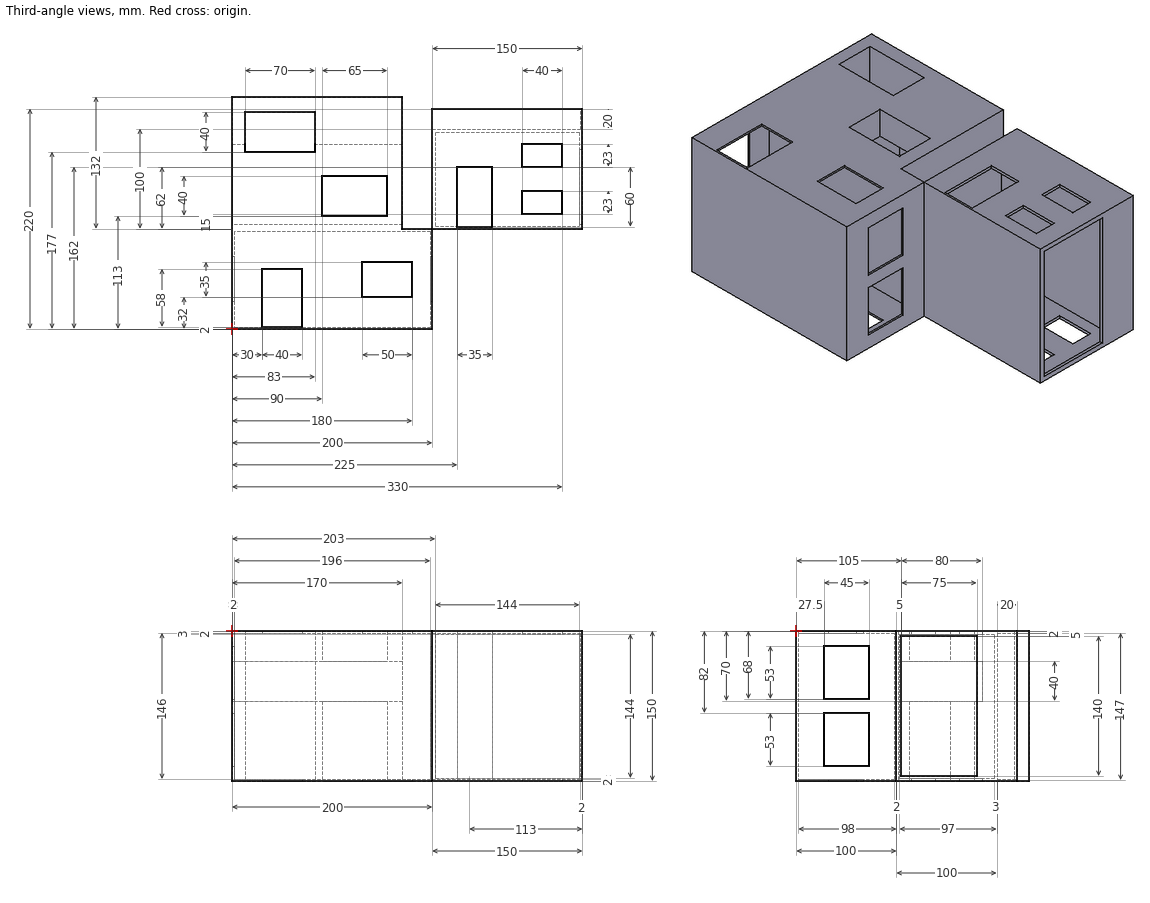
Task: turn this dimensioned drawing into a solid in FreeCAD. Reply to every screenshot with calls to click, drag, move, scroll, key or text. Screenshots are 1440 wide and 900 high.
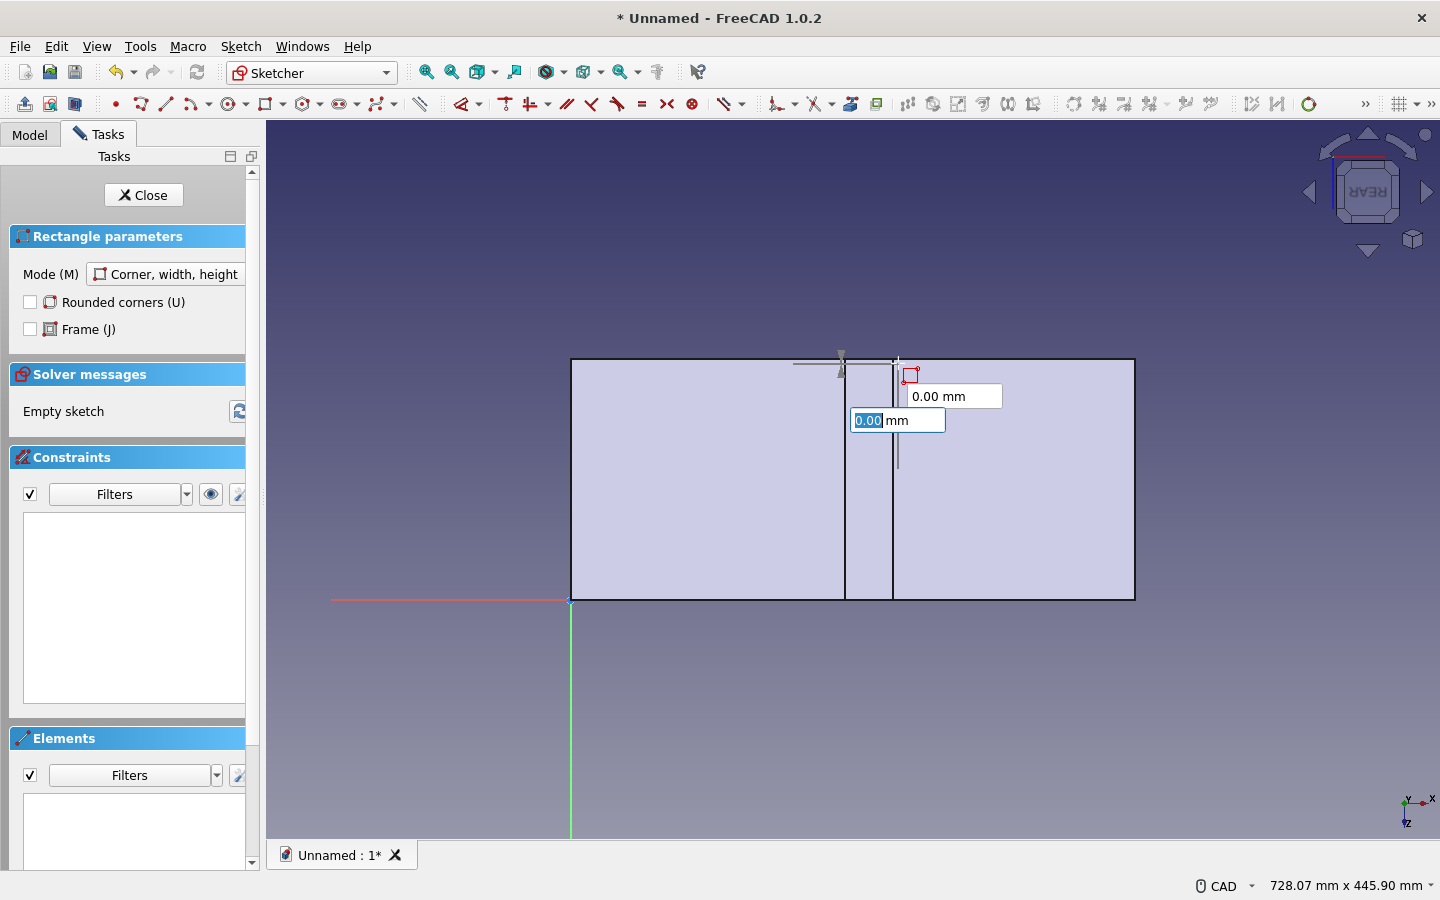
scroll(1130, 596, up, 6)
move(1129, 593)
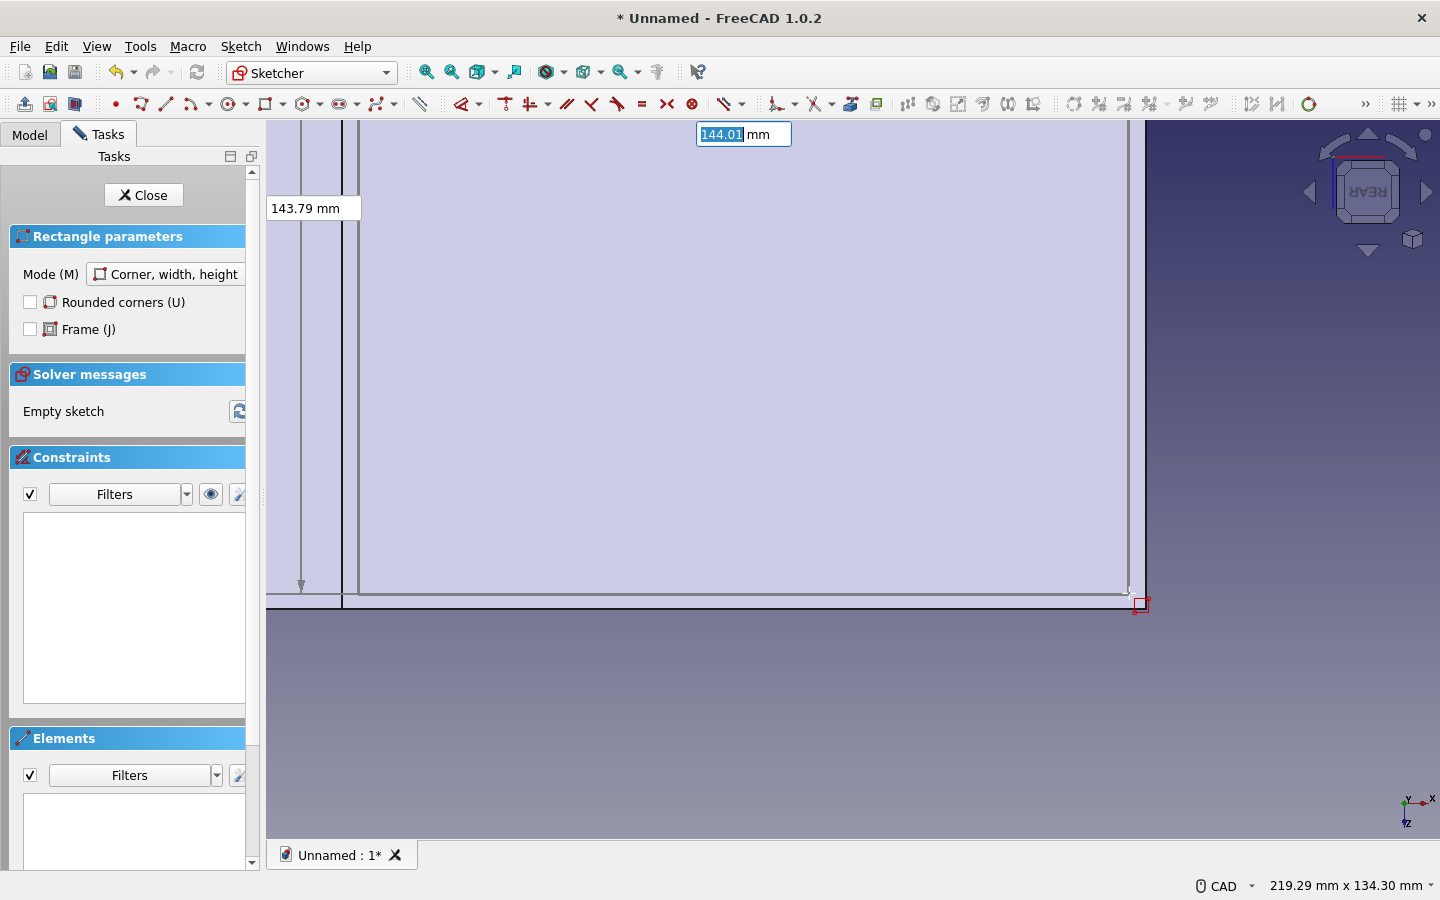
text(144)
key(Tab)
text(144)
key(Return)
key(Escape)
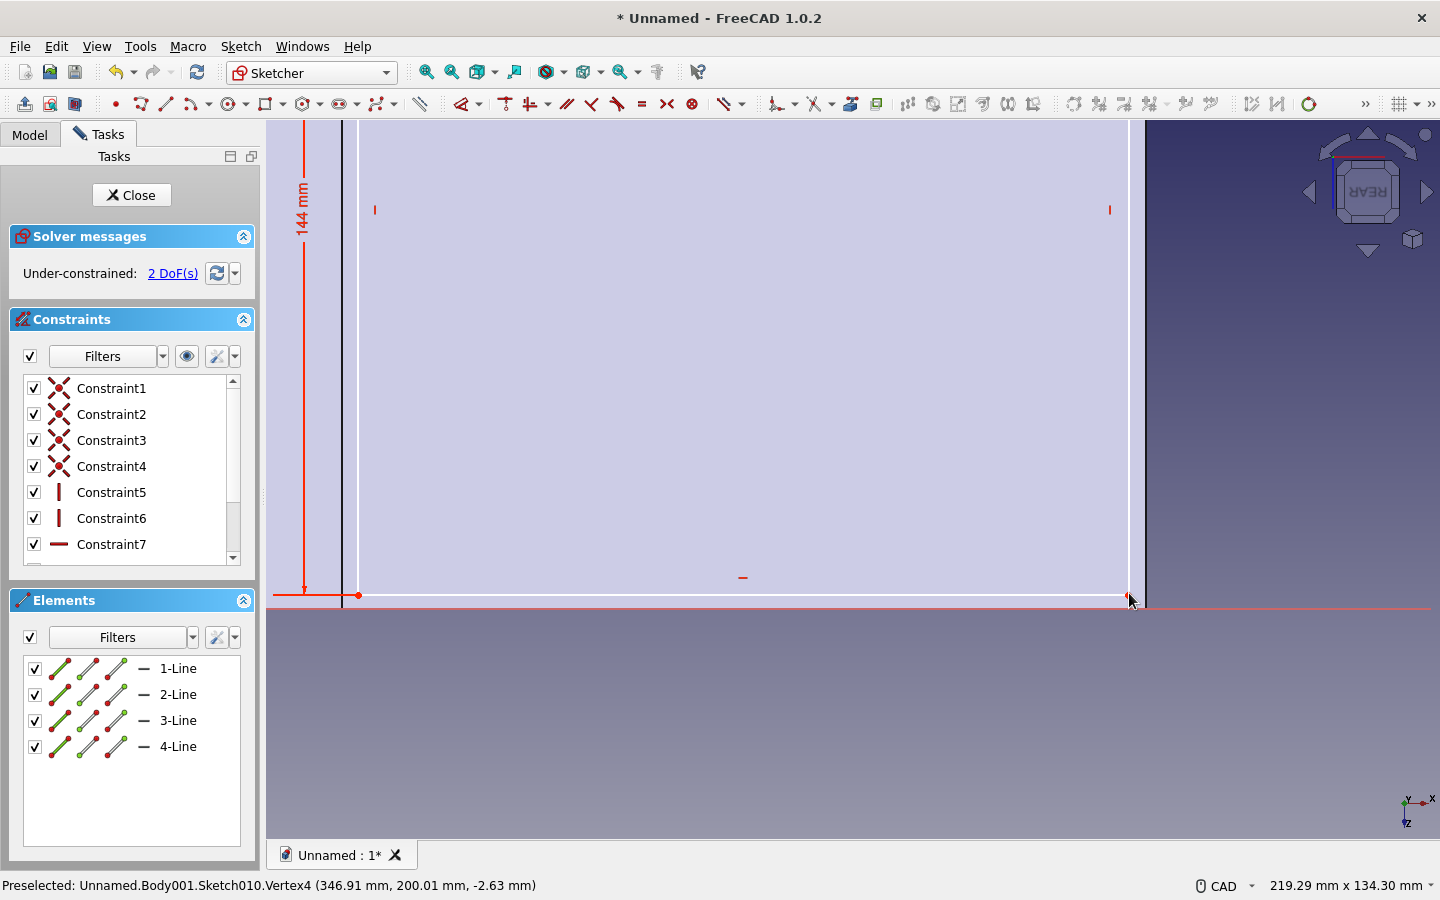
click(460, 104)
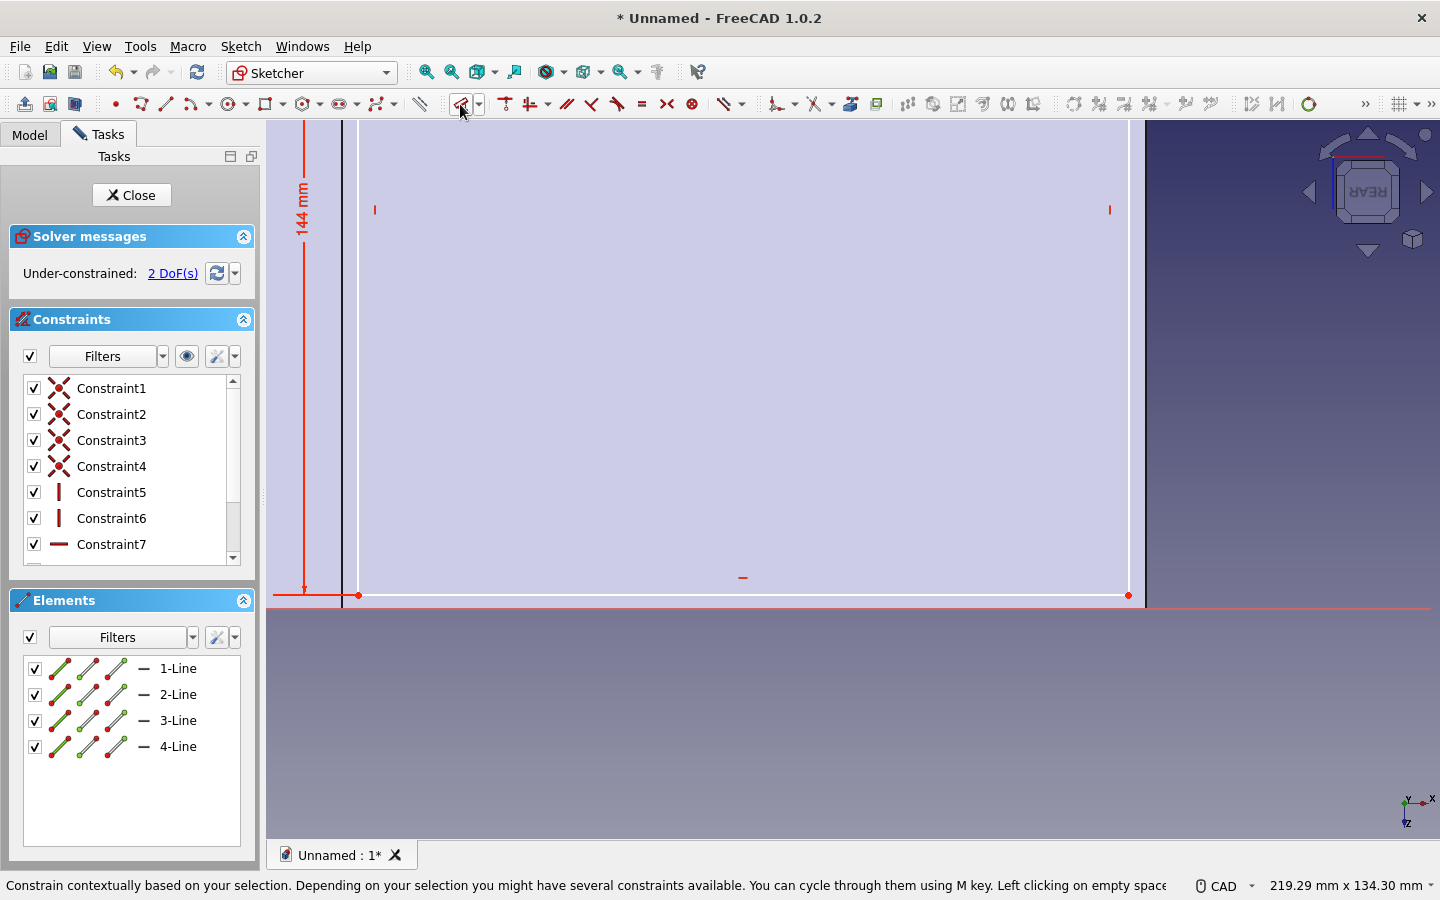
scroll(358, 595, up, 5)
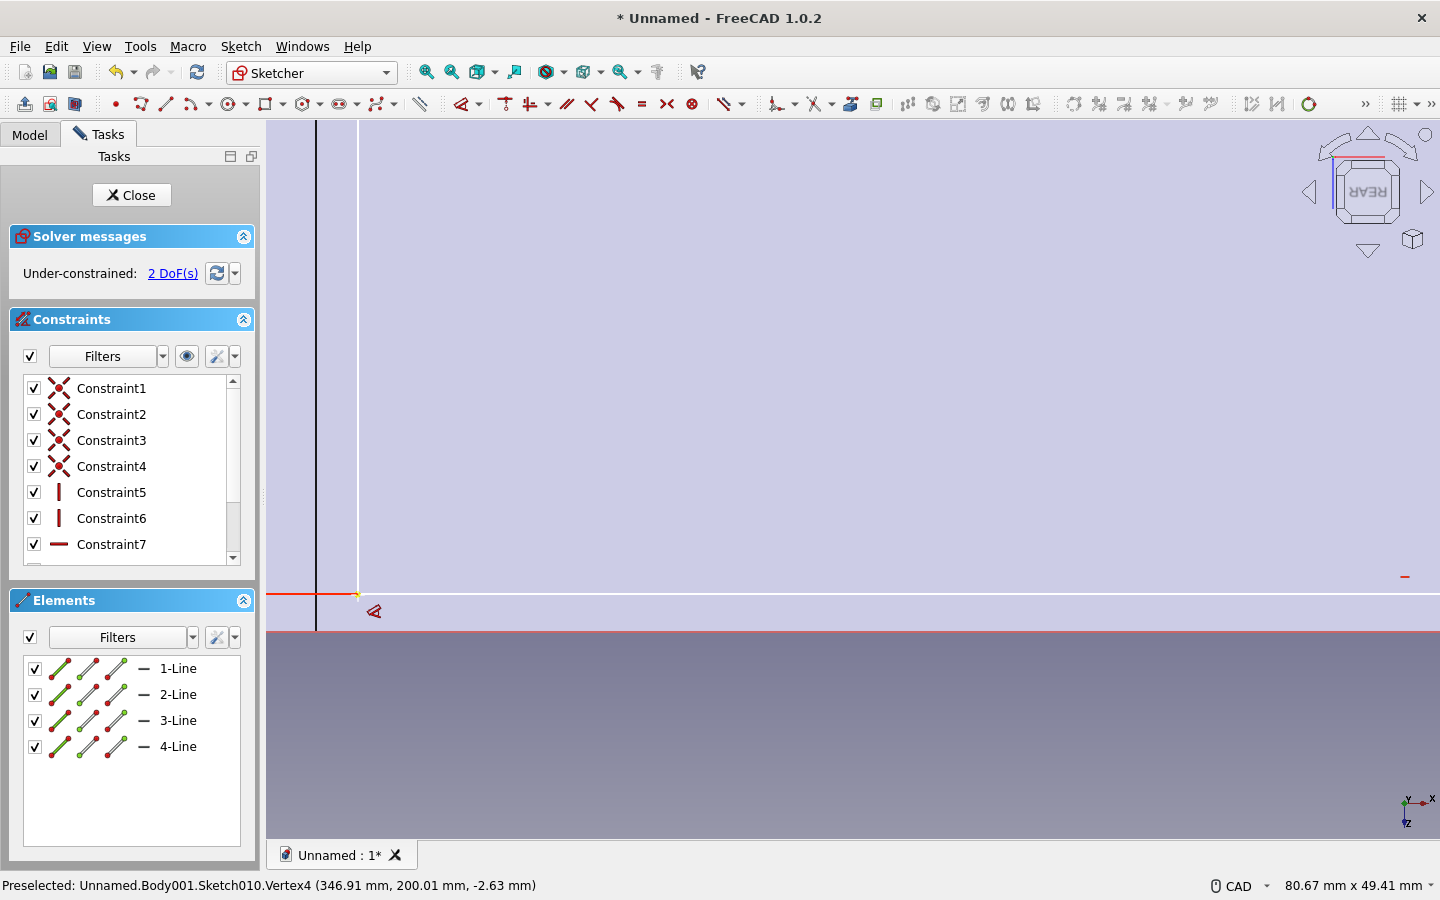
click(358, 594)
click(392, 613)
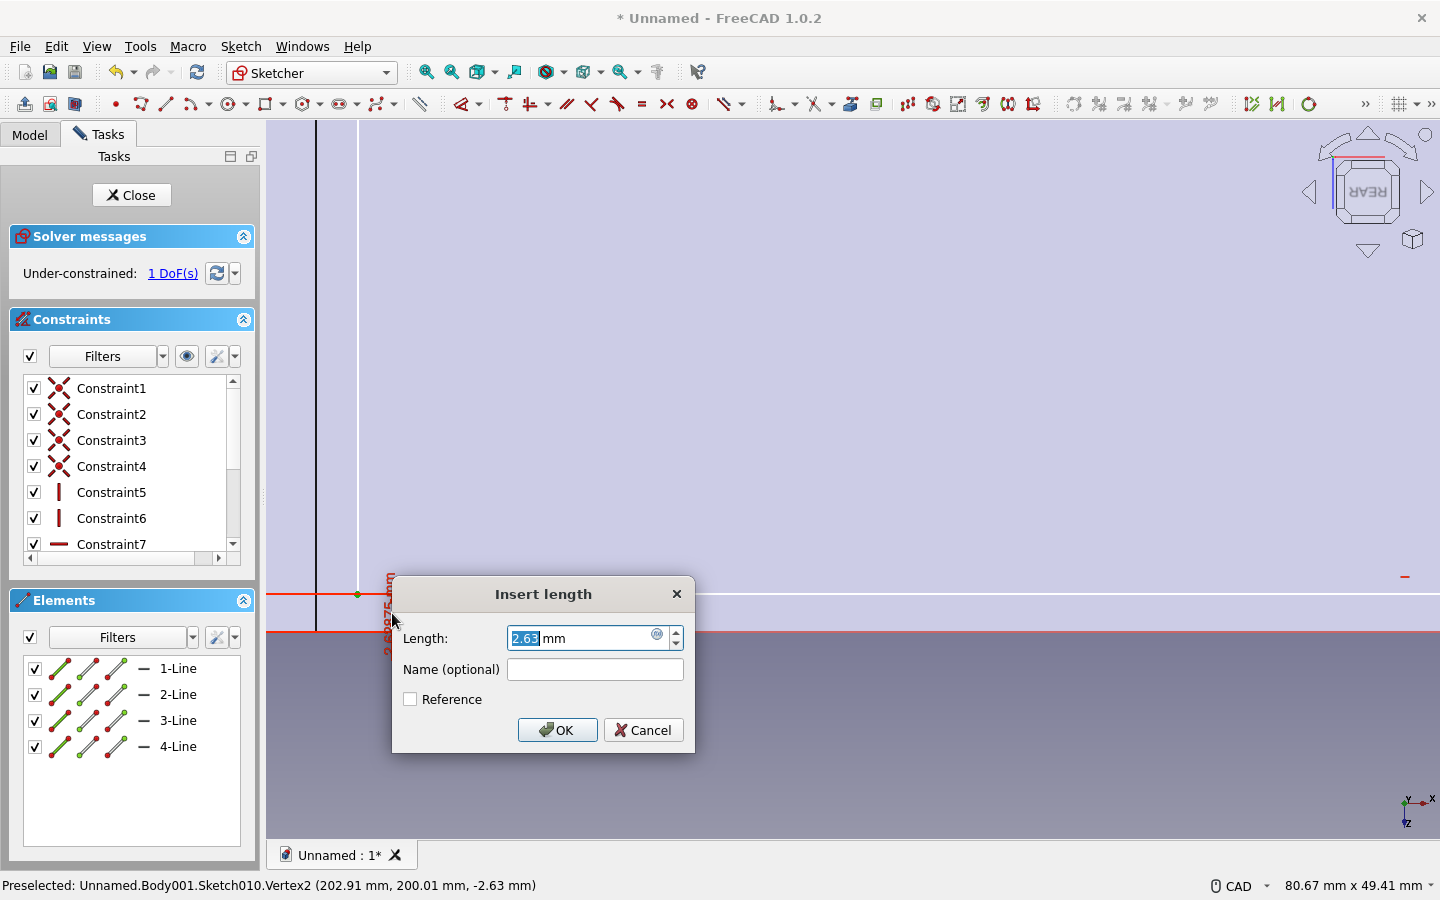
text(3)
key(Return)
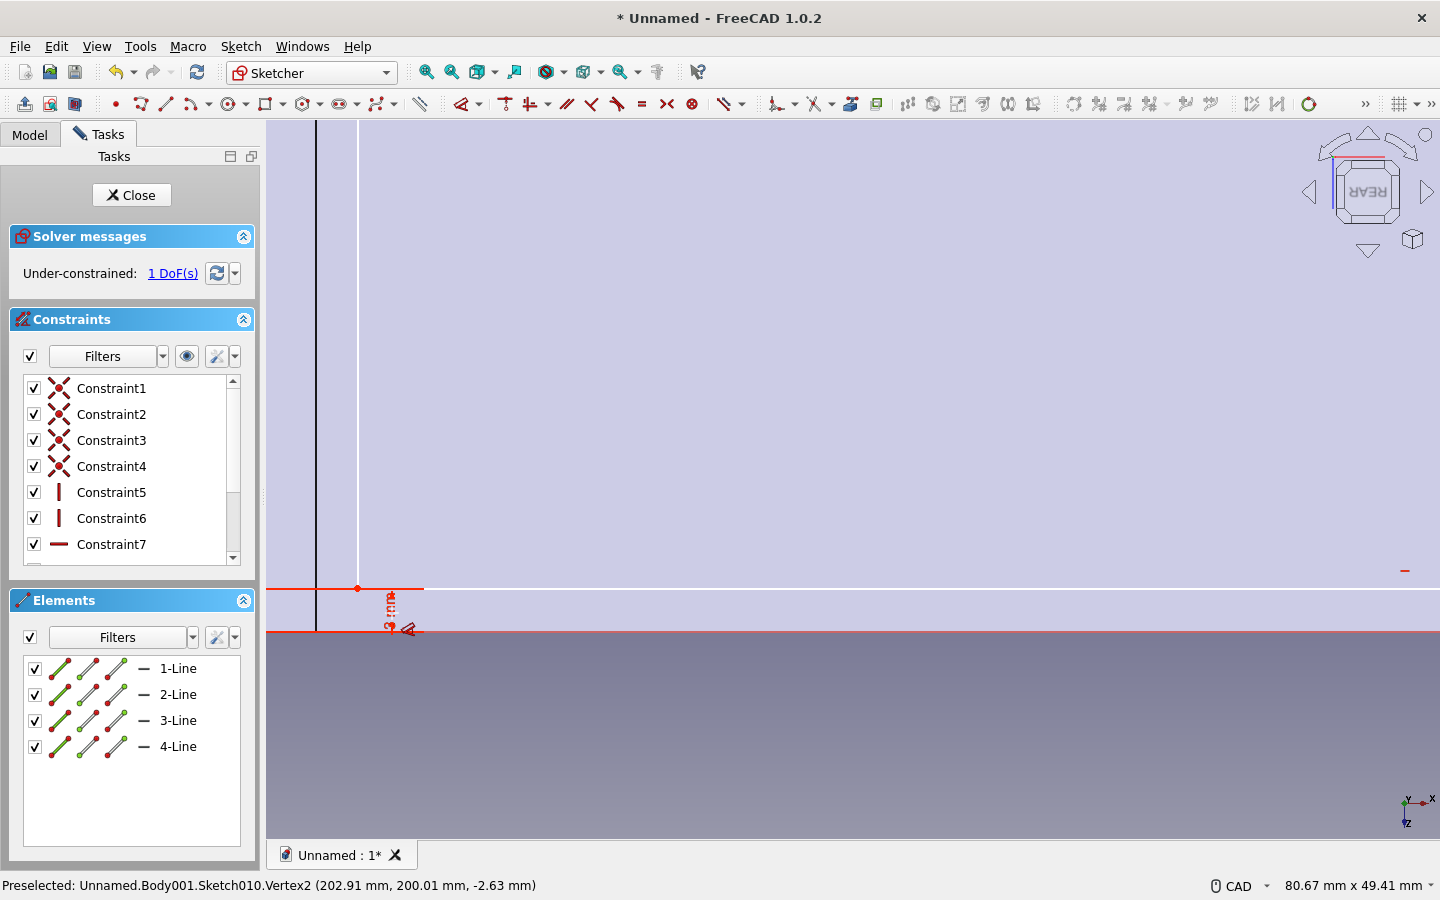
scroll(918, 623, down, 10)